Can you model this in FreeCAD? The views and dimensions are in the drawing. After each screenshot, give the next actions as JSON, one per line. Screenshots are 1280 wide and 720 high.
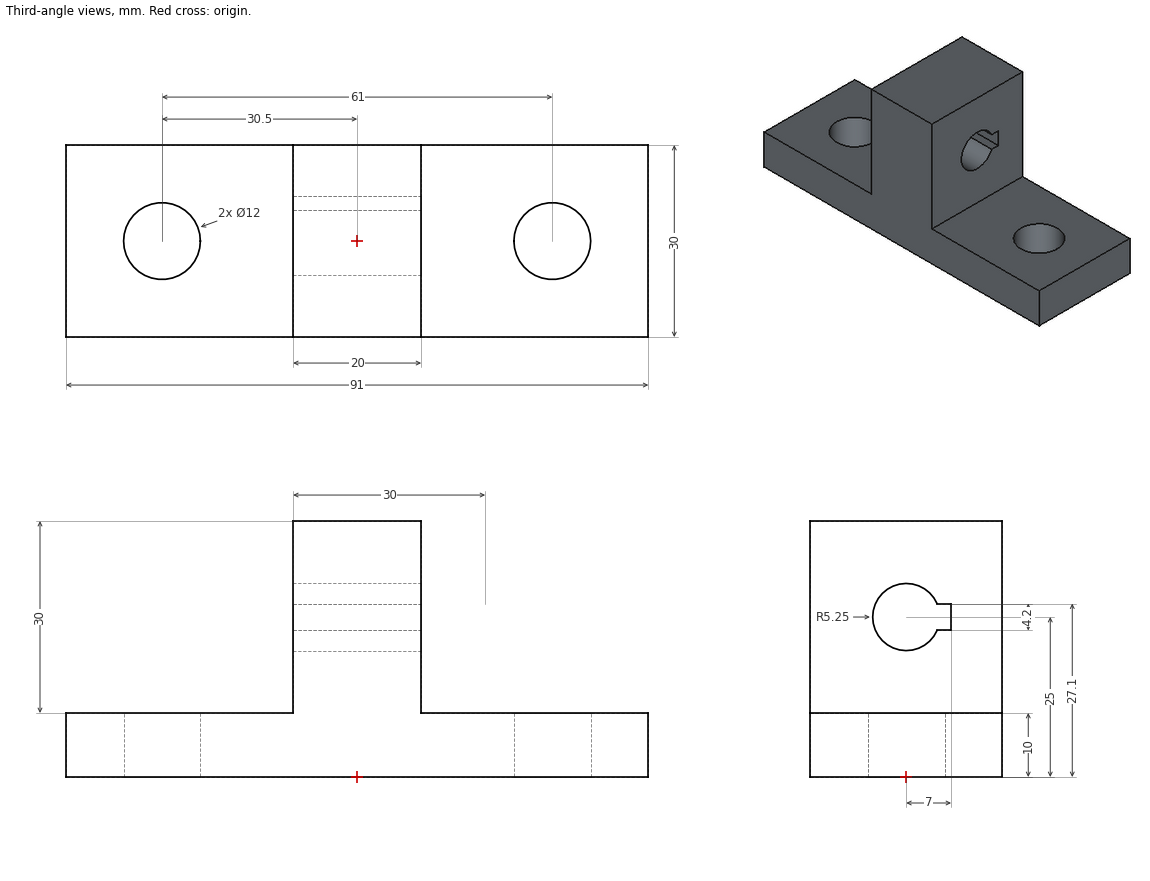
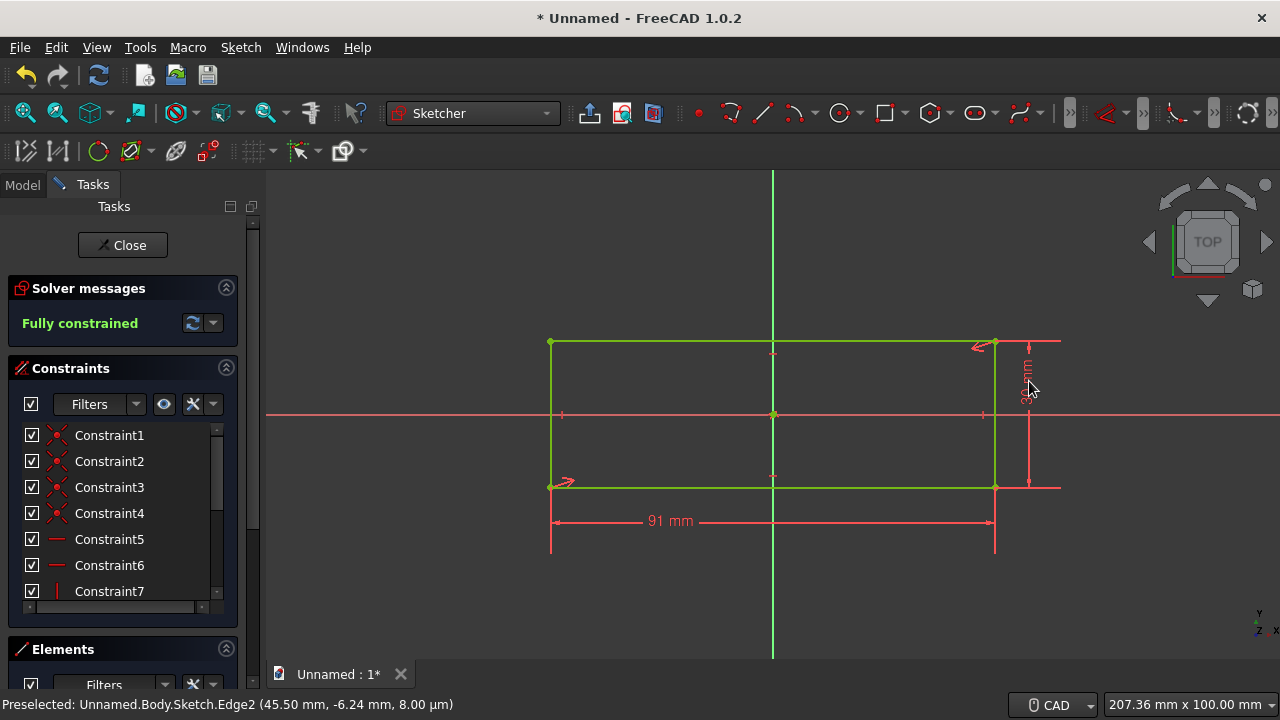
{"action": "left_click", "coordinate": [123, 245]}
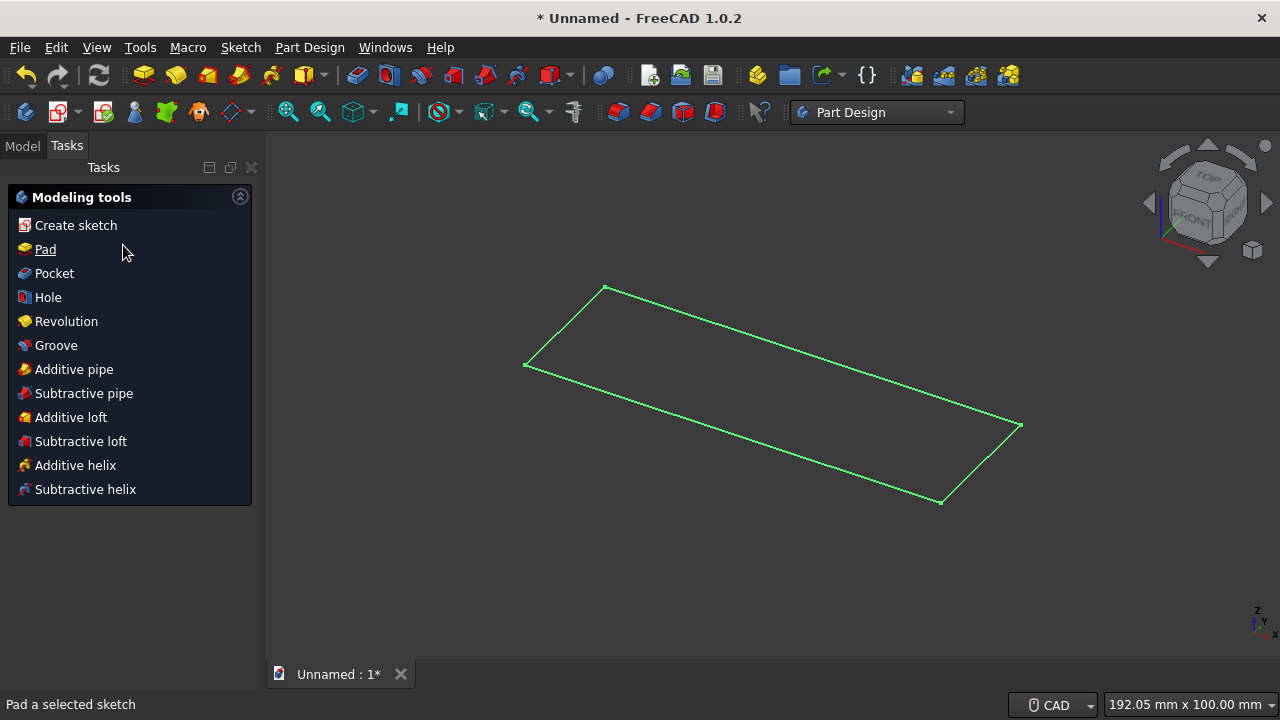
{"action": "left_click", "coordinate": [144, 76]}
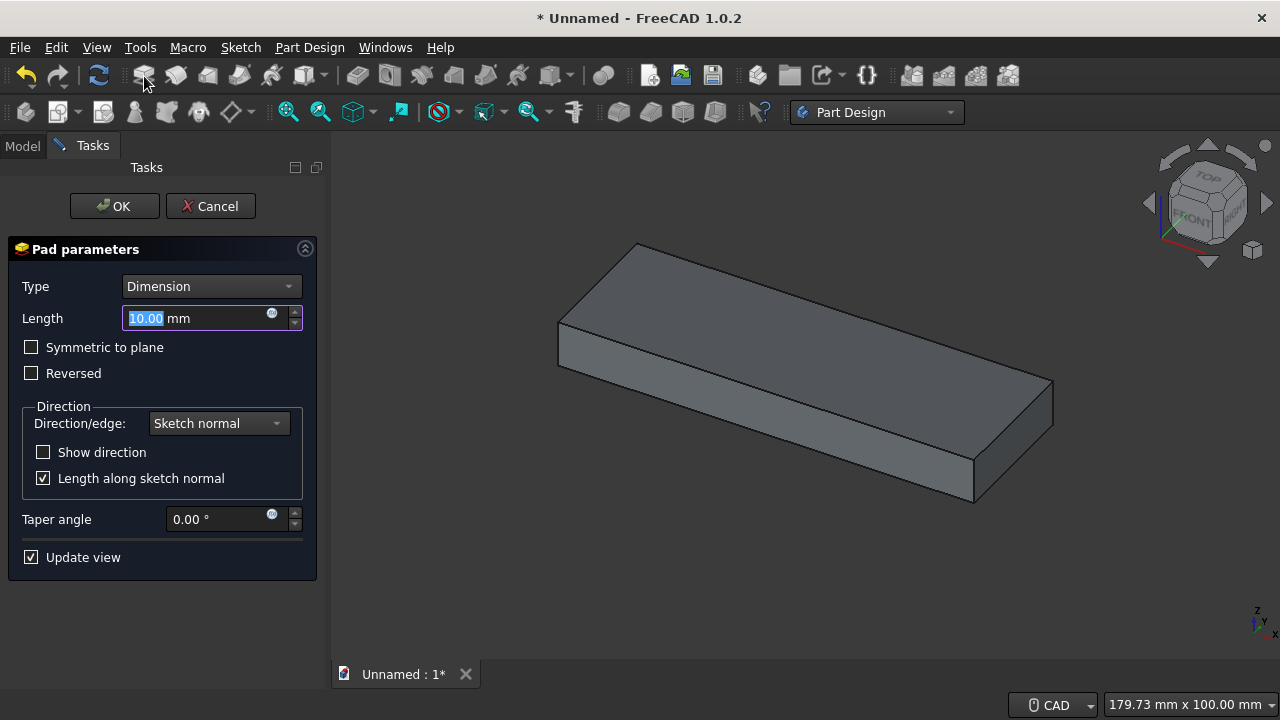
{"action": "type", "text": "10"}
{"action": "key", "text": "Tab"}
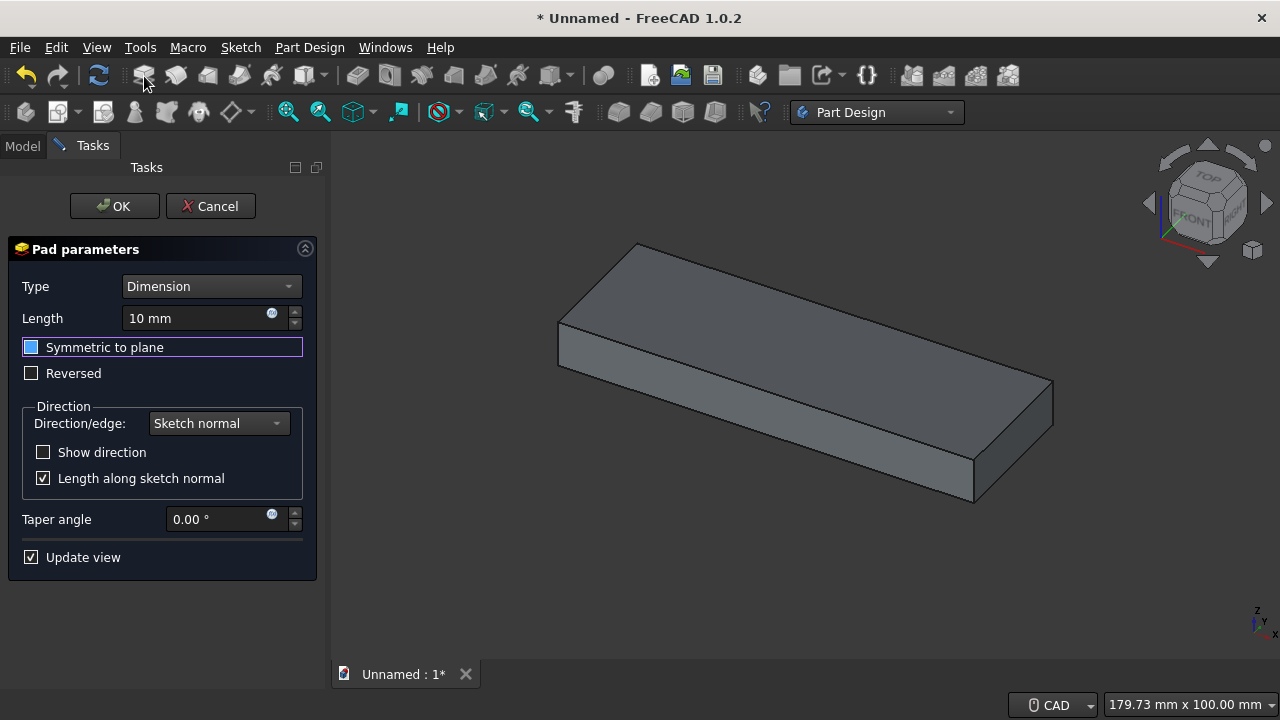
{"action": "left_click", "coordinate": [115, 206]}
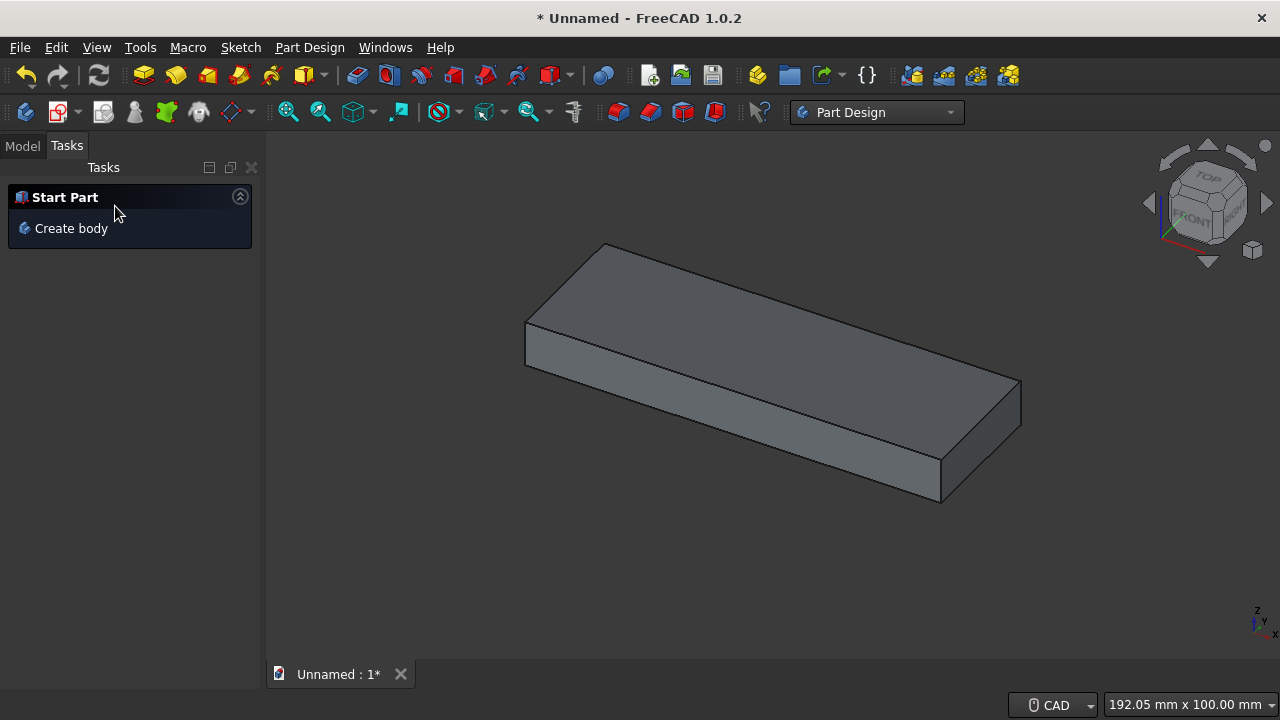
{"action": "left_click", "coordinate": [892, 390]}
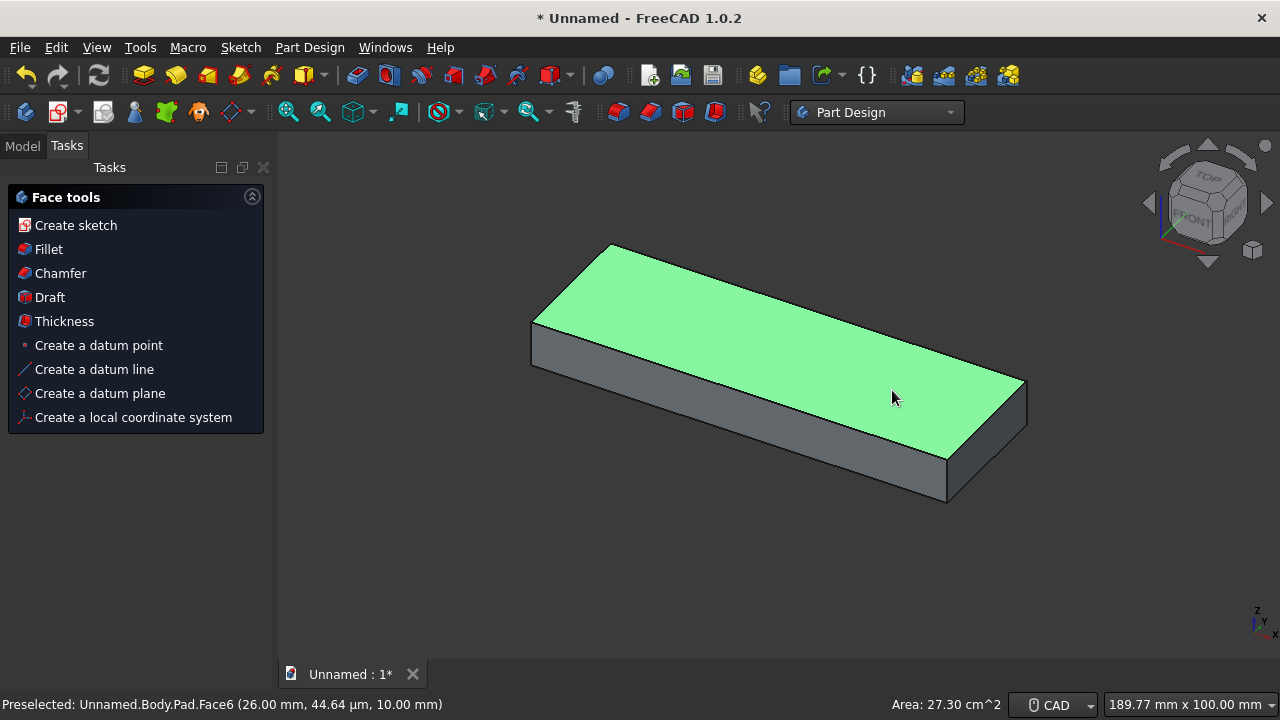
{"action": "left_click", "coordinate": [58, 112]}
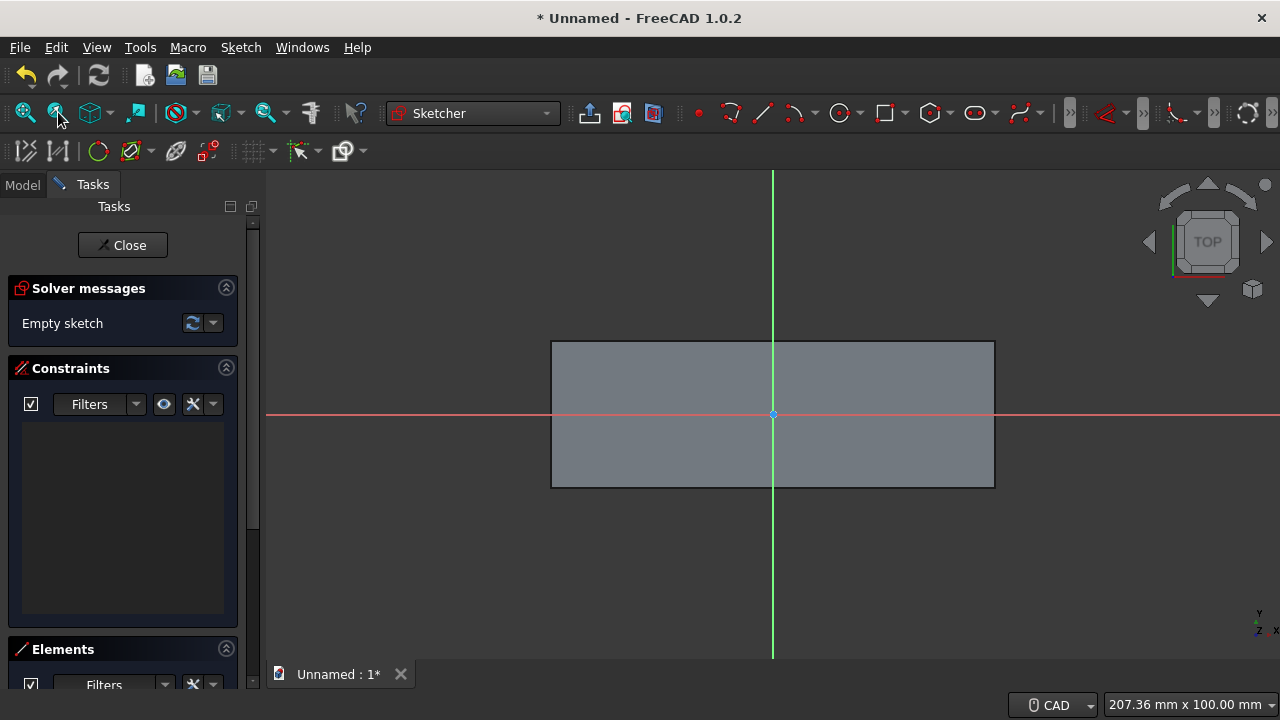
{"action": "scroll", "coordinate": [829, 414], "scroll_direction": "up", "scroll_amount": 4}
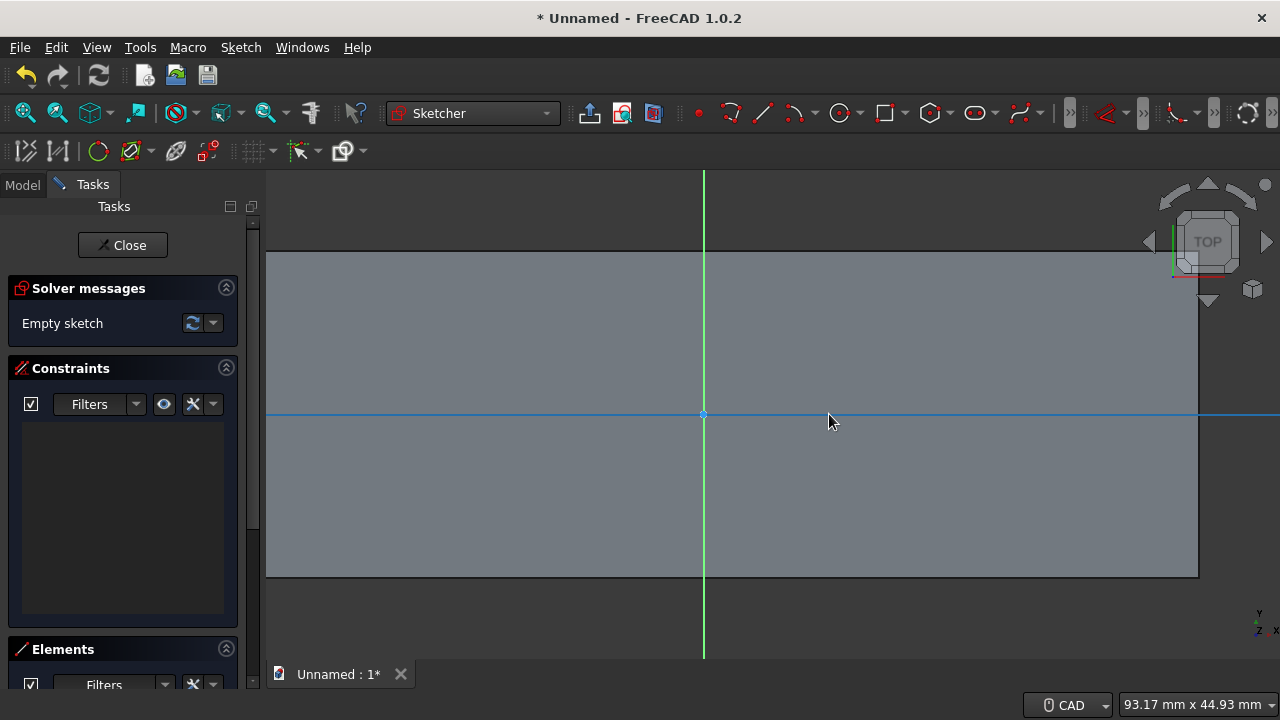
{"action": "key", "text": "g v"}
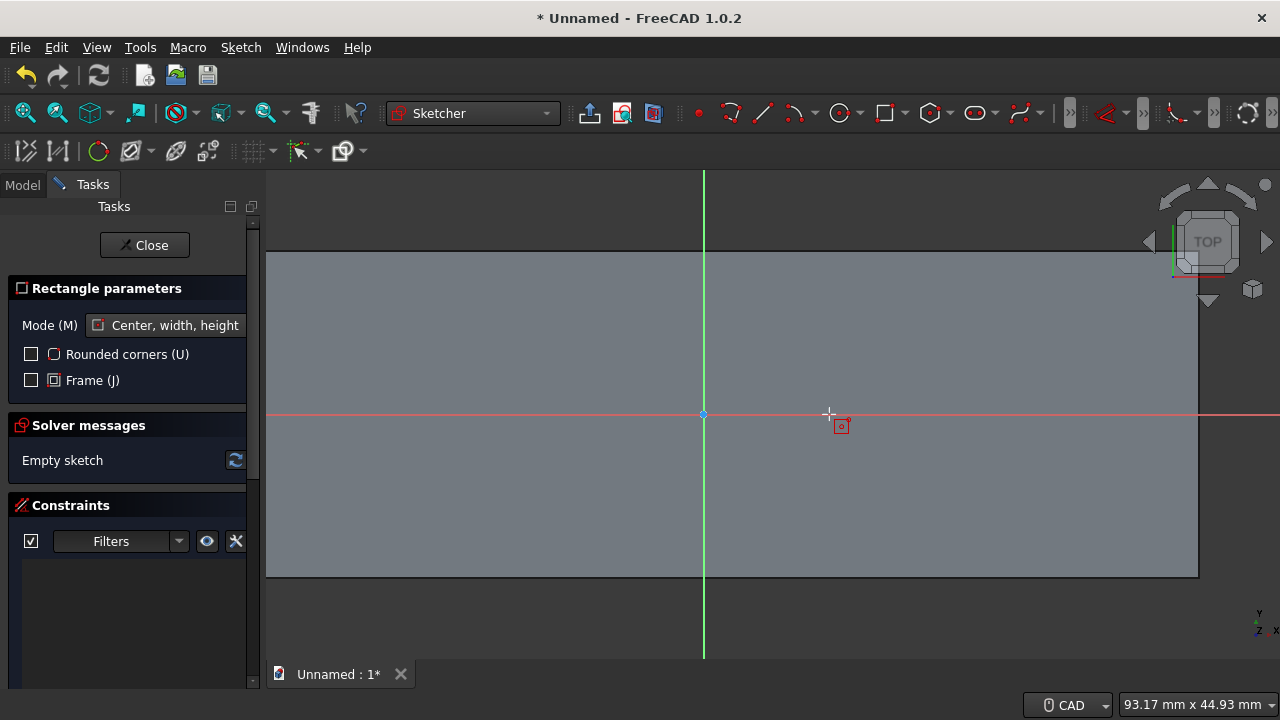
{"action": "left_click", "coordinate": [704, 414]}
{"action": "left_click", "coordinate": [813, 251]}
{"action": "key", "text": "Escape"}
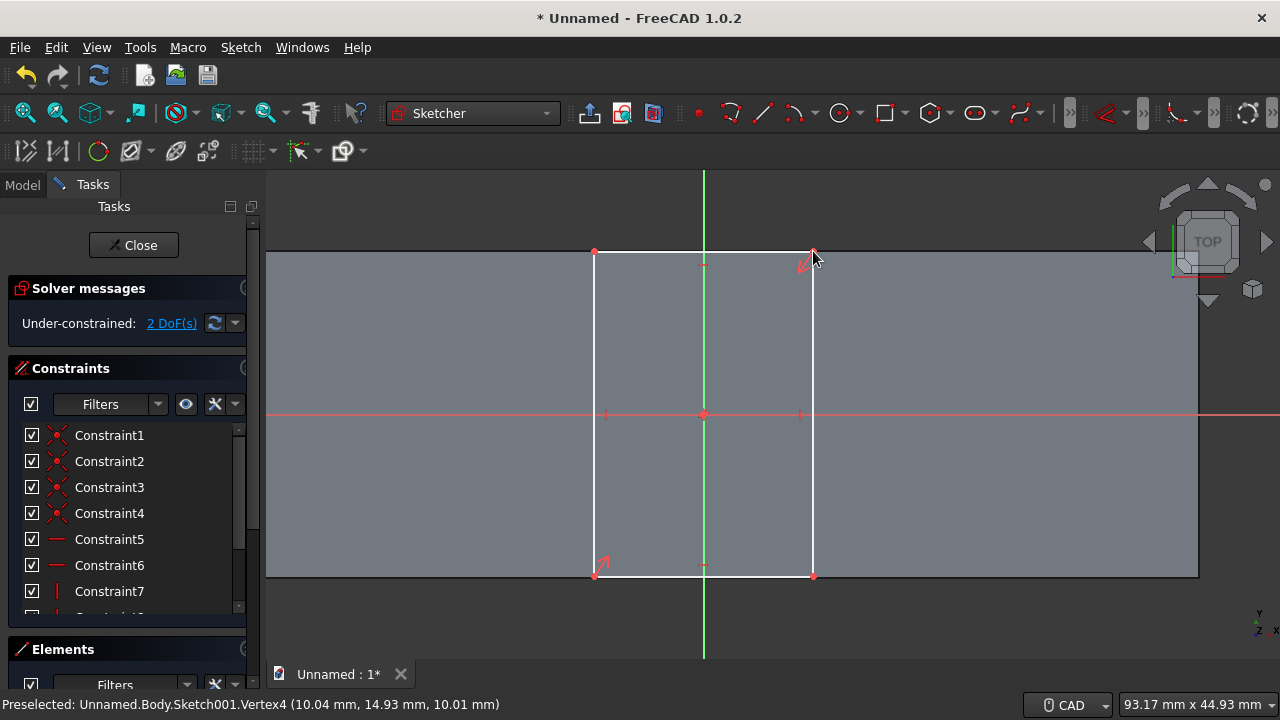
{"action": "key", "text": "d"}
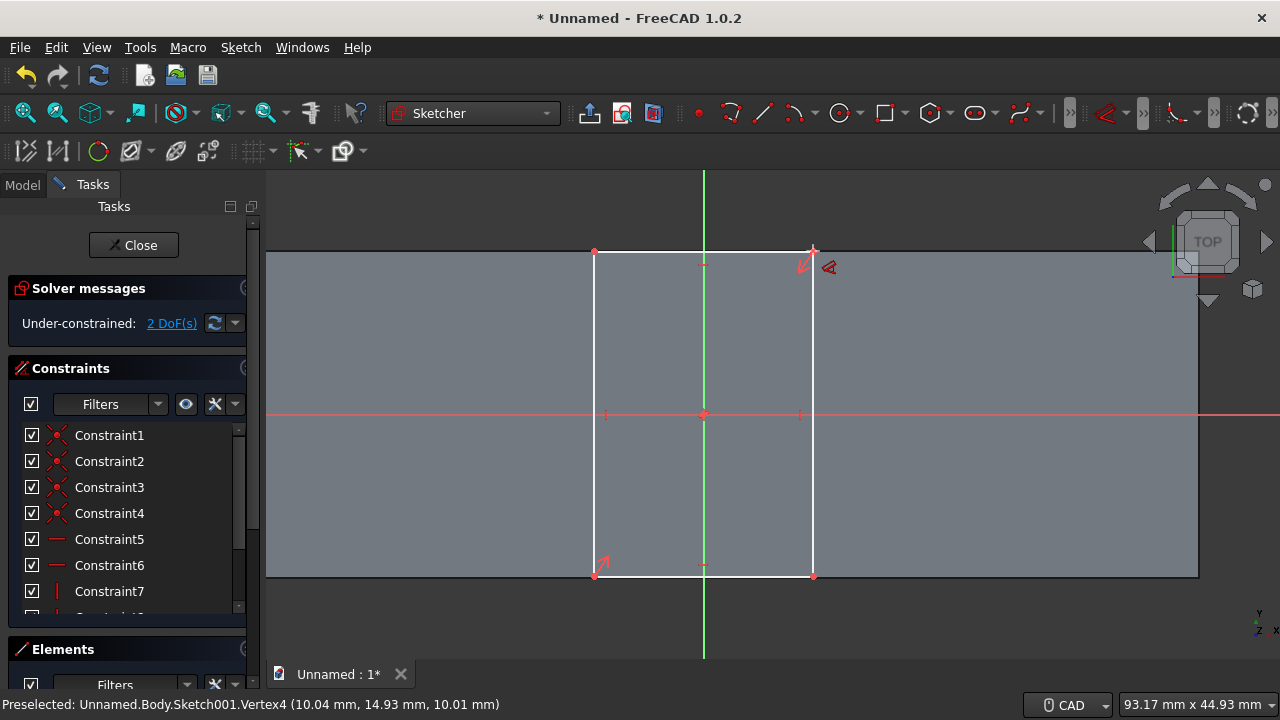
{"action": "left_click", "coordinate": [660, 577]}
{"action": "left_click", "coordinate": [653, 611]}